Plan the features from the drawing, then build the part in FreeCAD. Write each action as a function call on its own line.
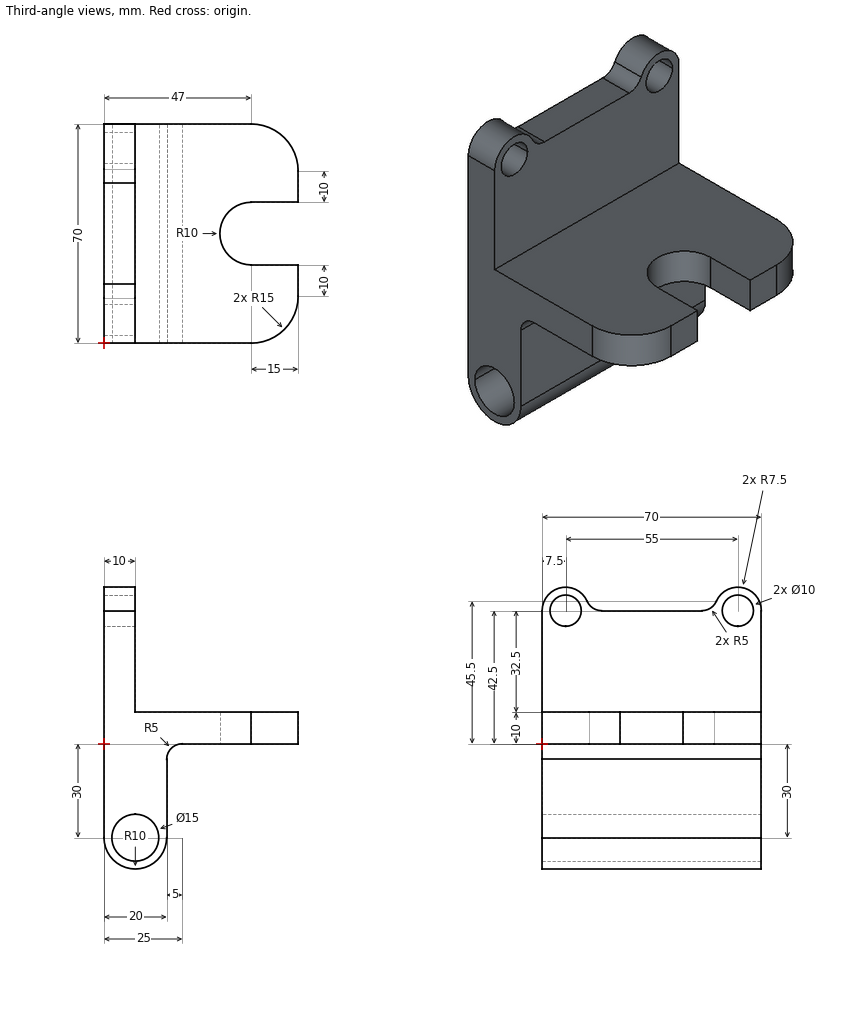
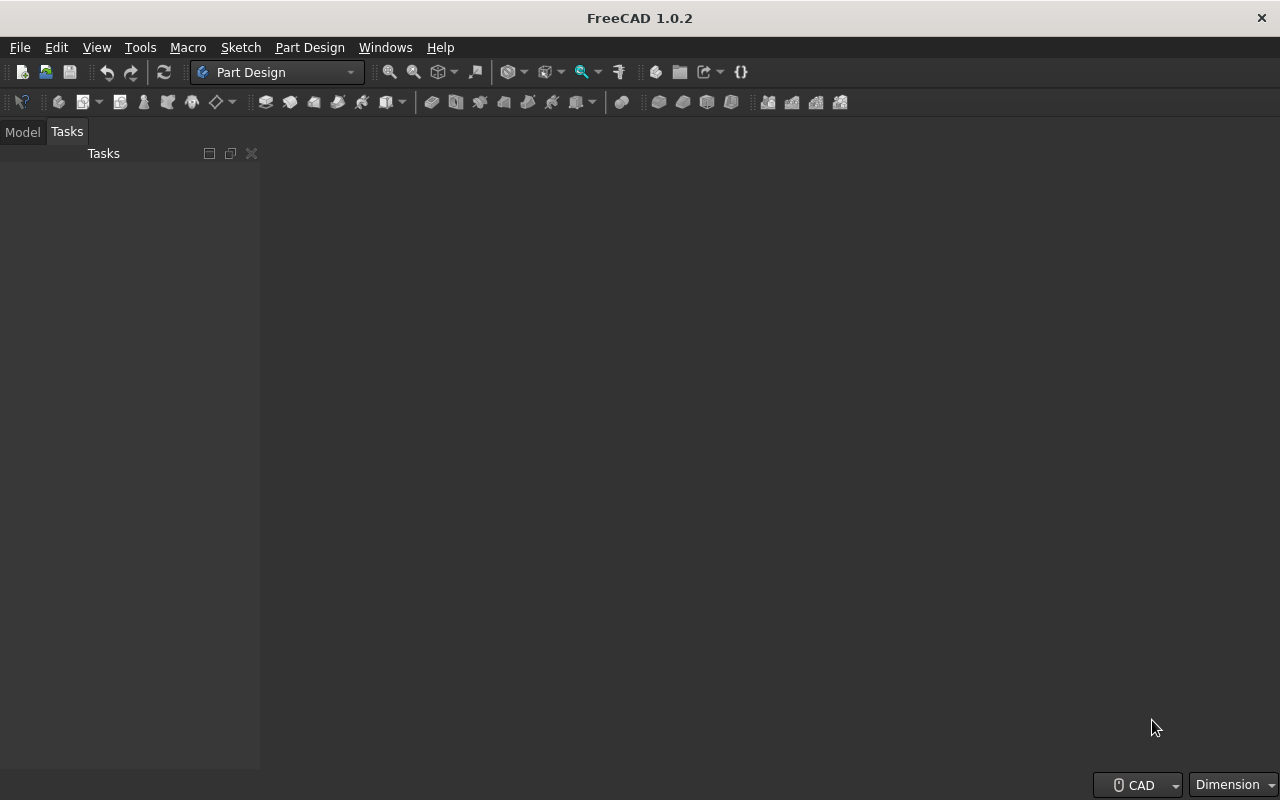
click(22, 72)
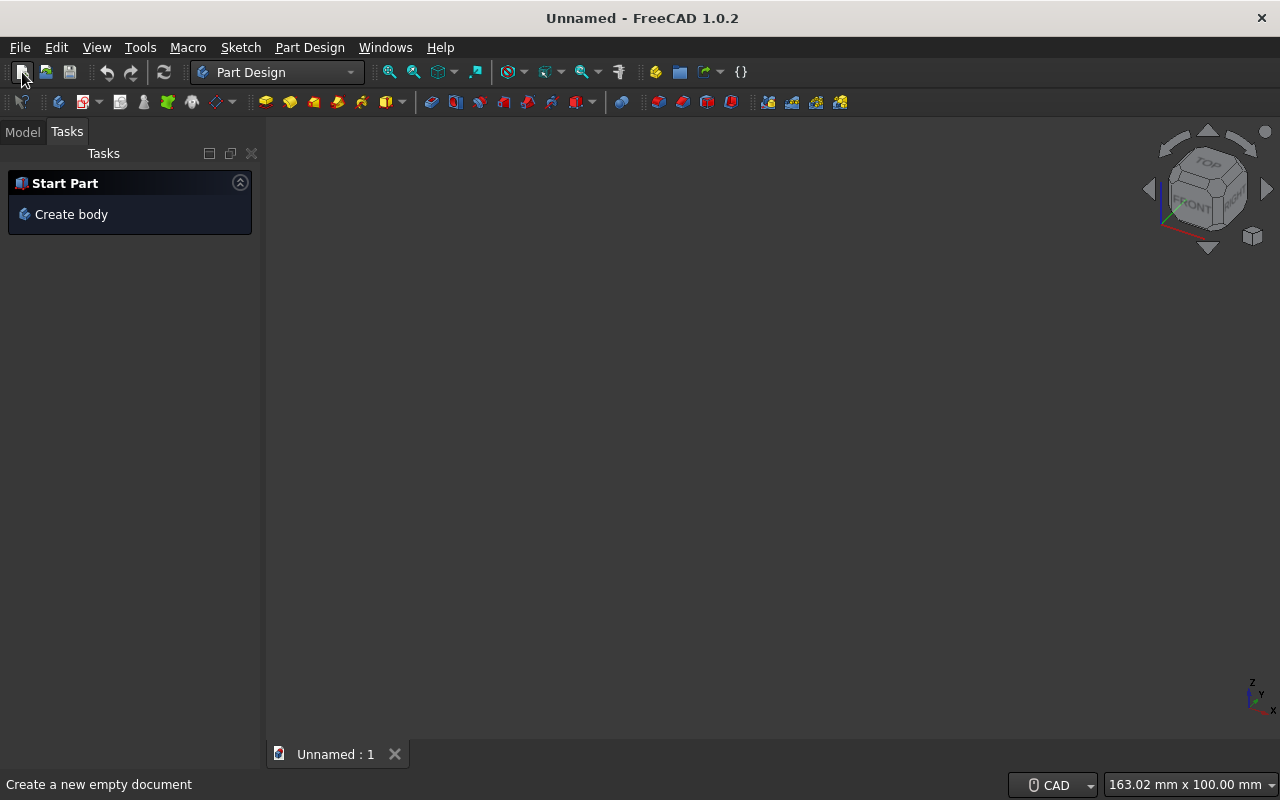
click(84, 102)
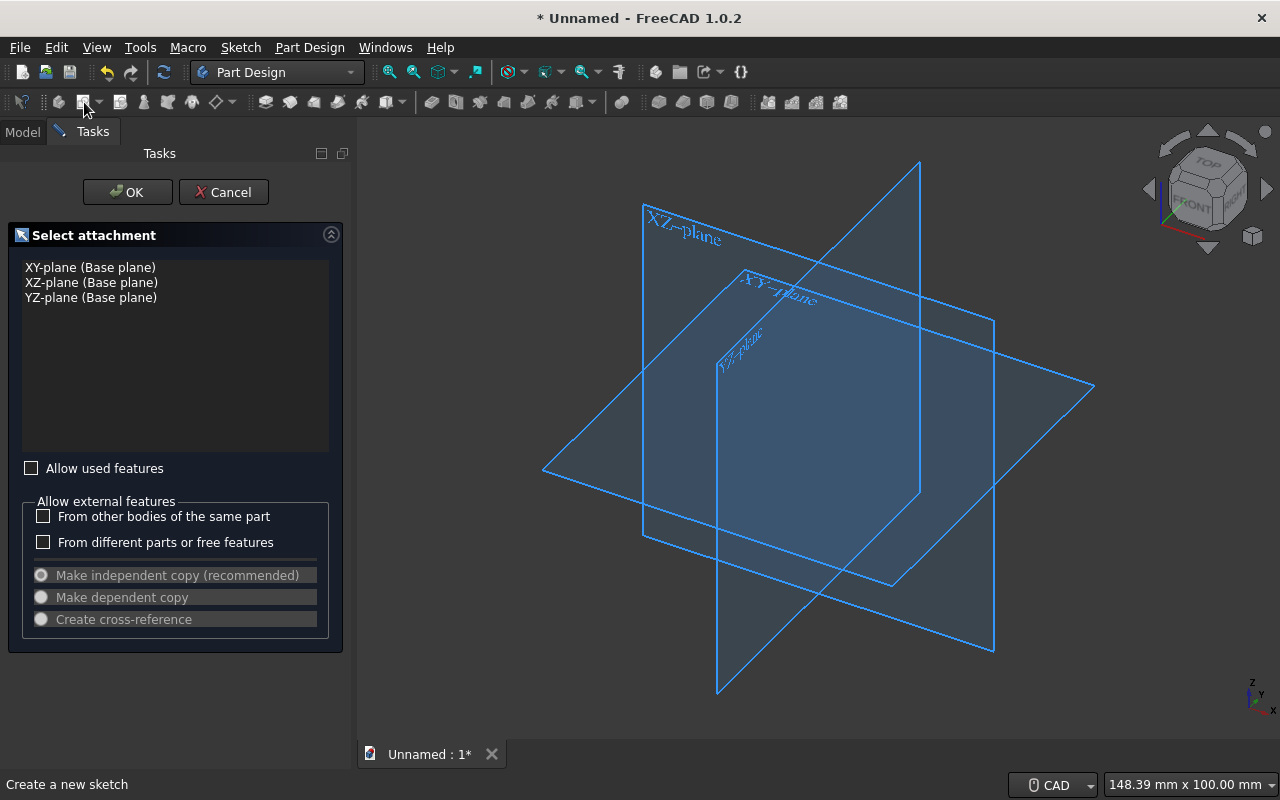
click(82, 268)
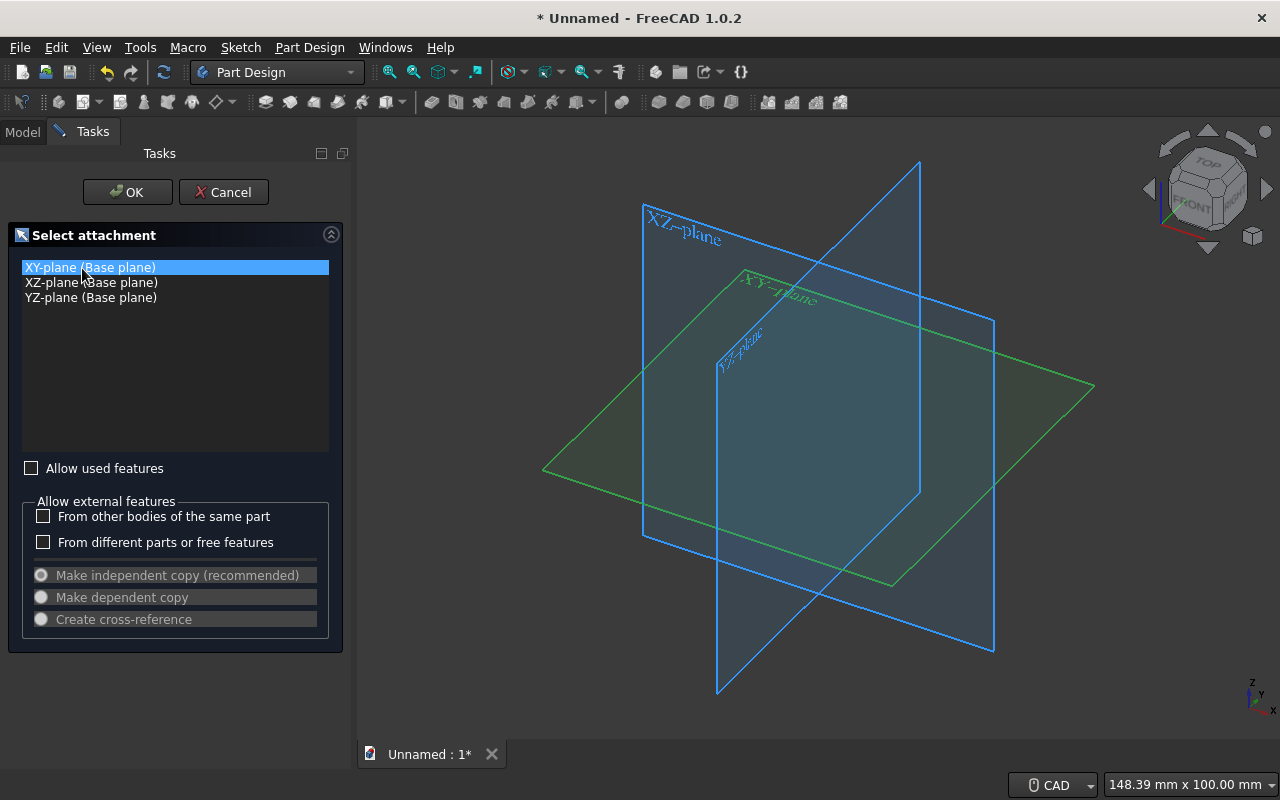
click(128, 192)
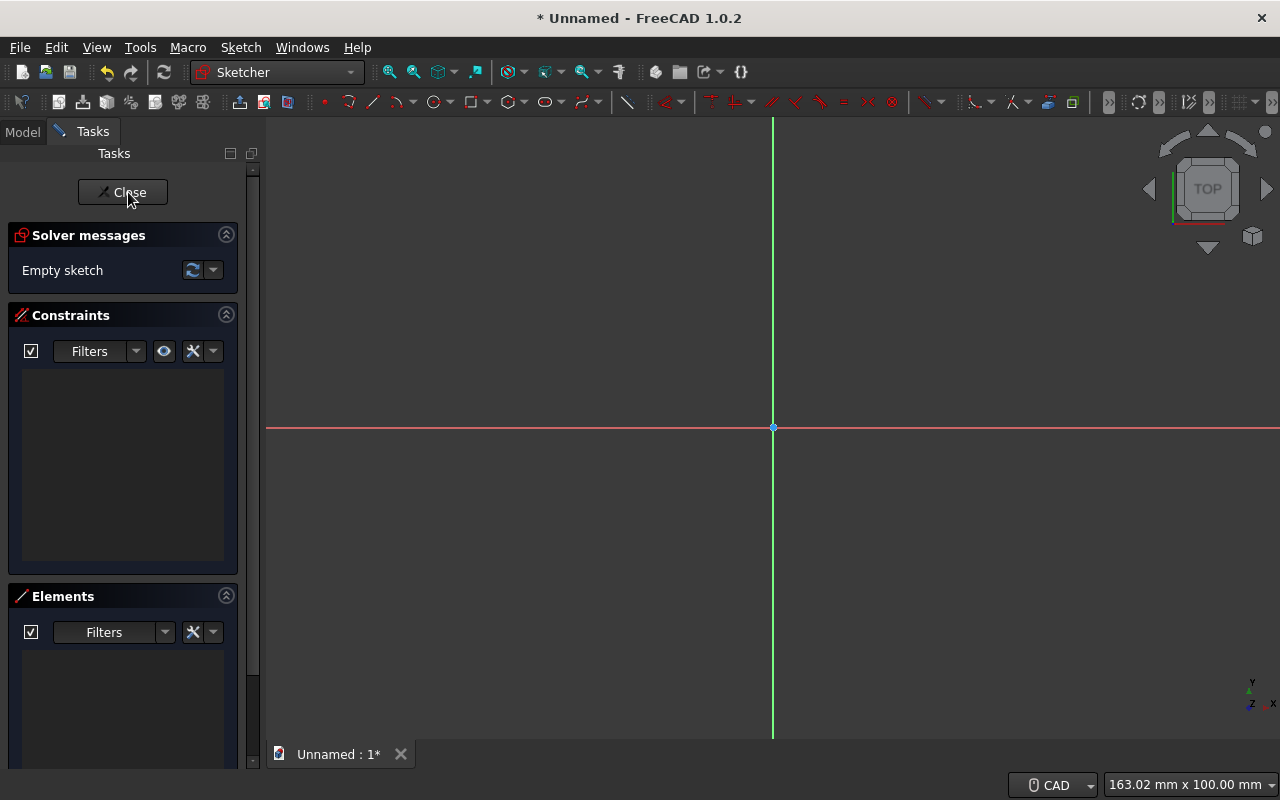
scroll(294, 711, down, 2)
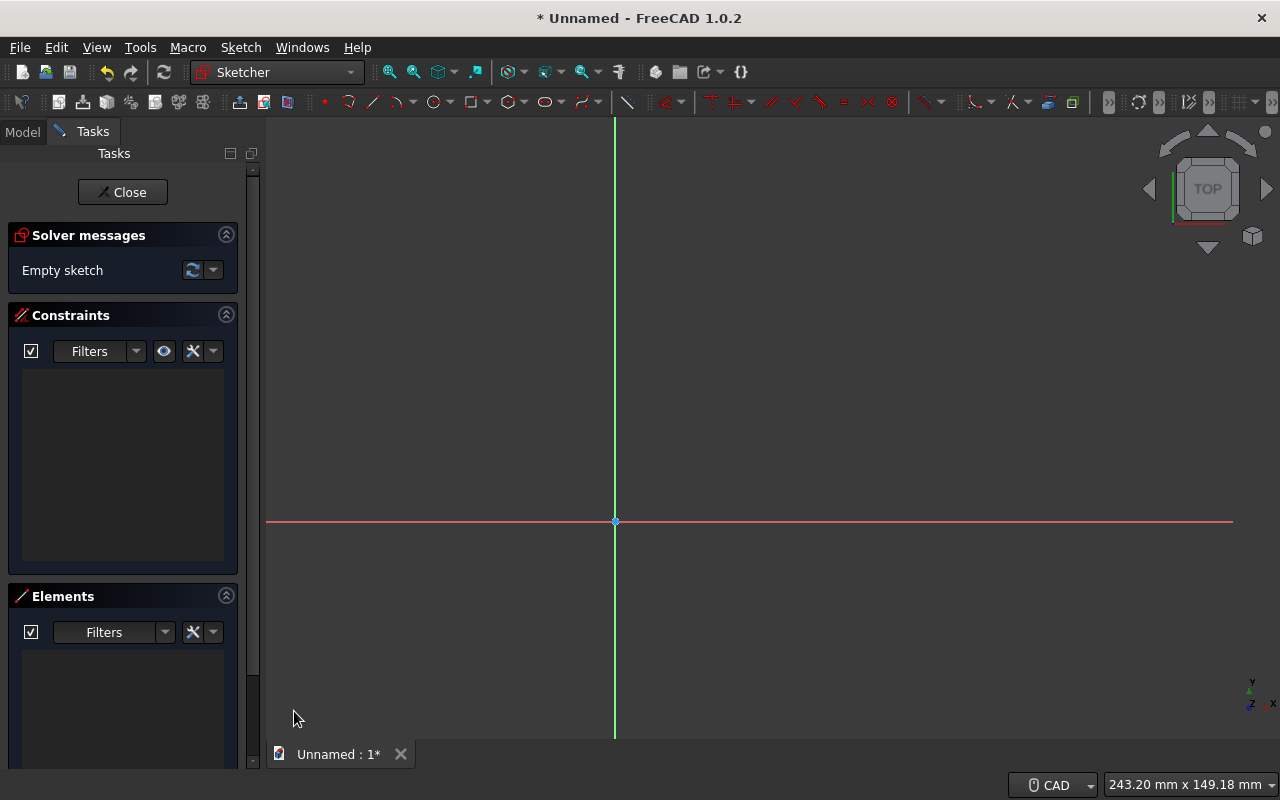
scroll(825, 269, up, 2)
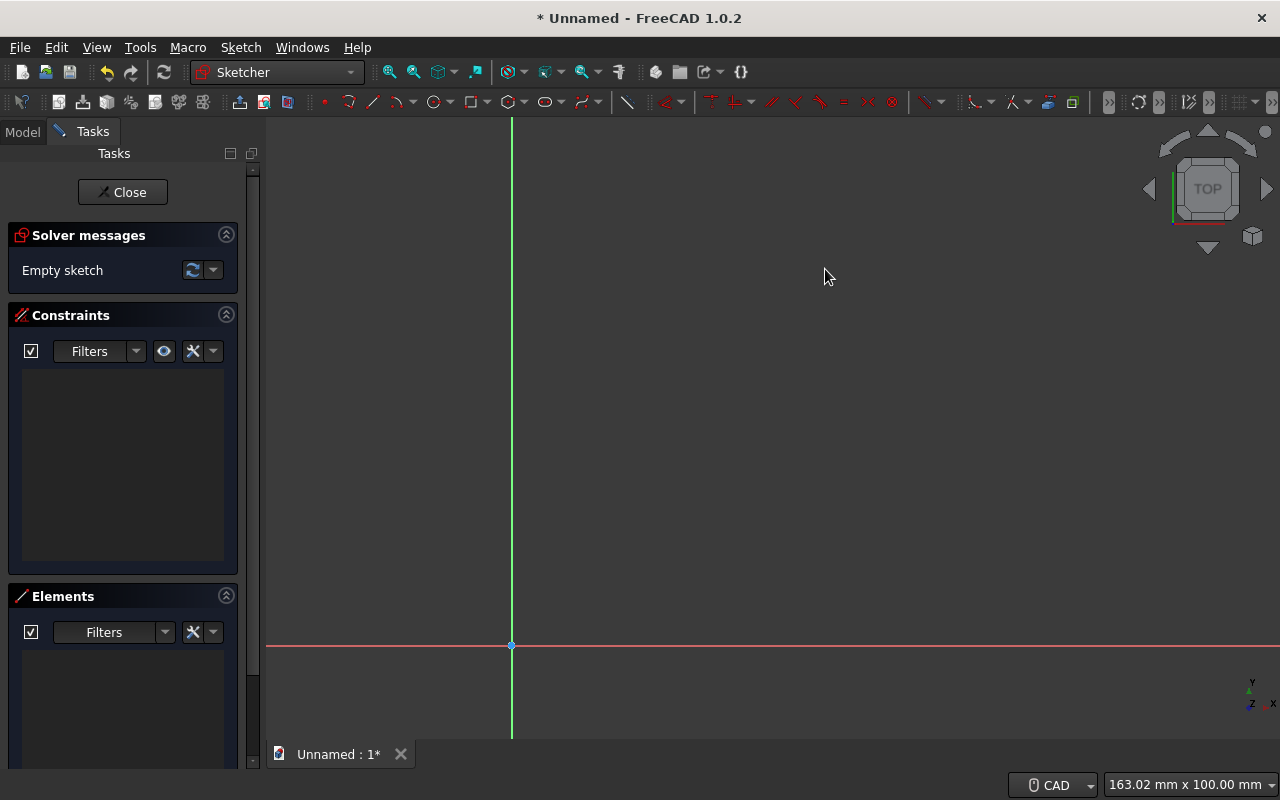
click(350, 102)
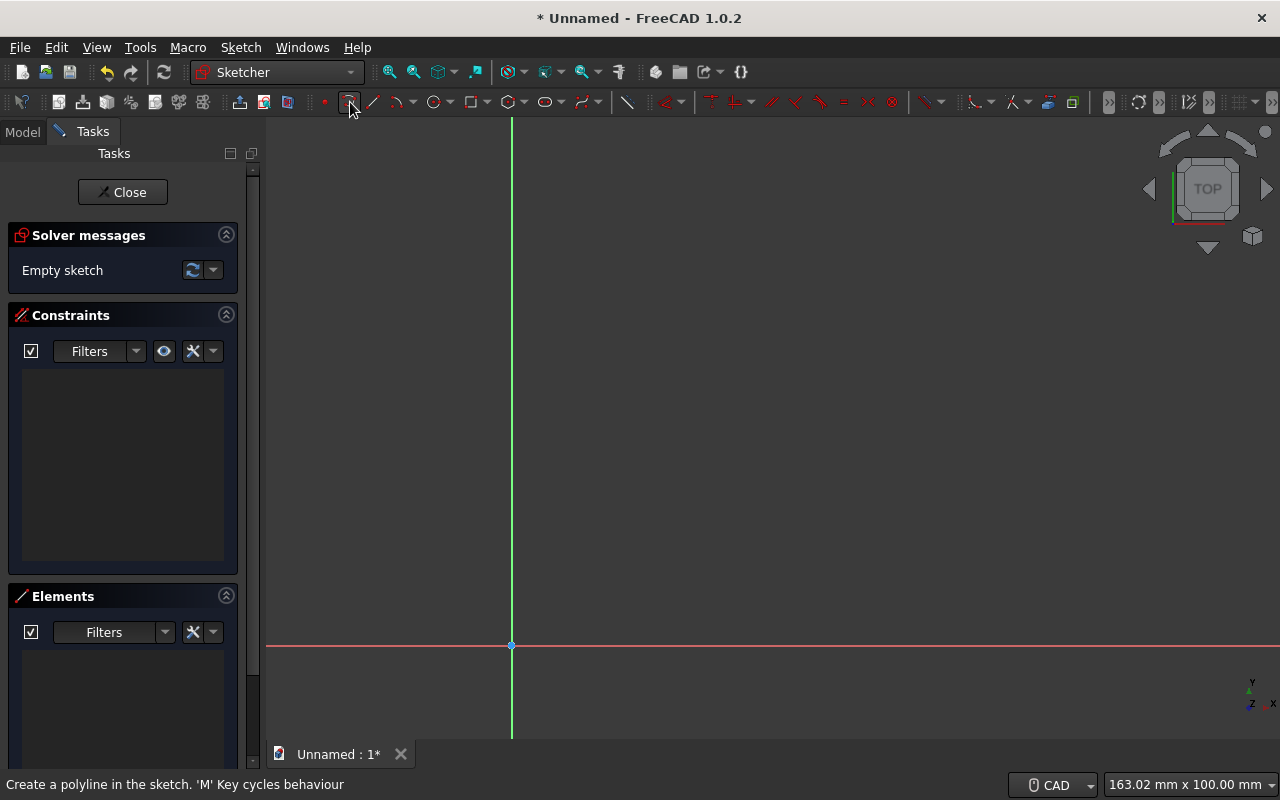
click(897, 552)
click(897, 490)
click(804, 490)
right_click(804, 490)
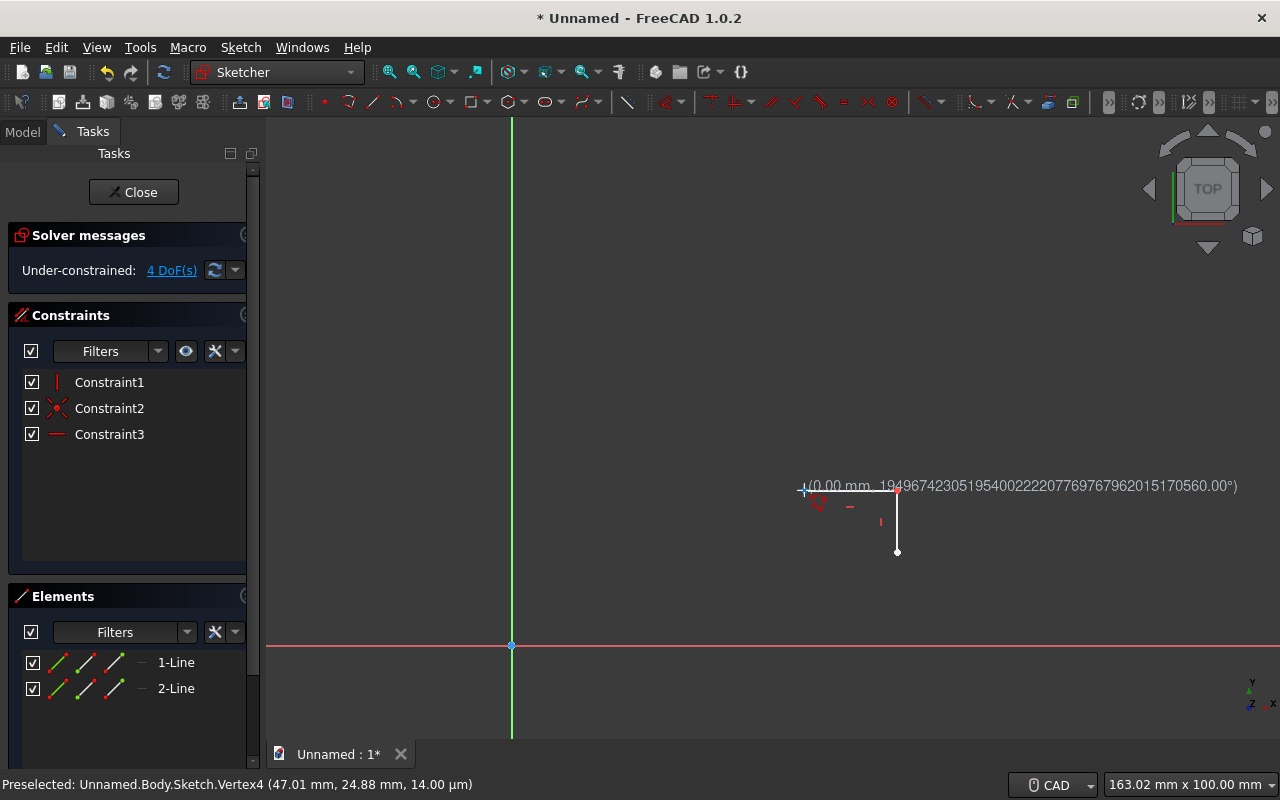
click(804, 366)
click(897, 366)
click(897, 304)
right_click(897, 304)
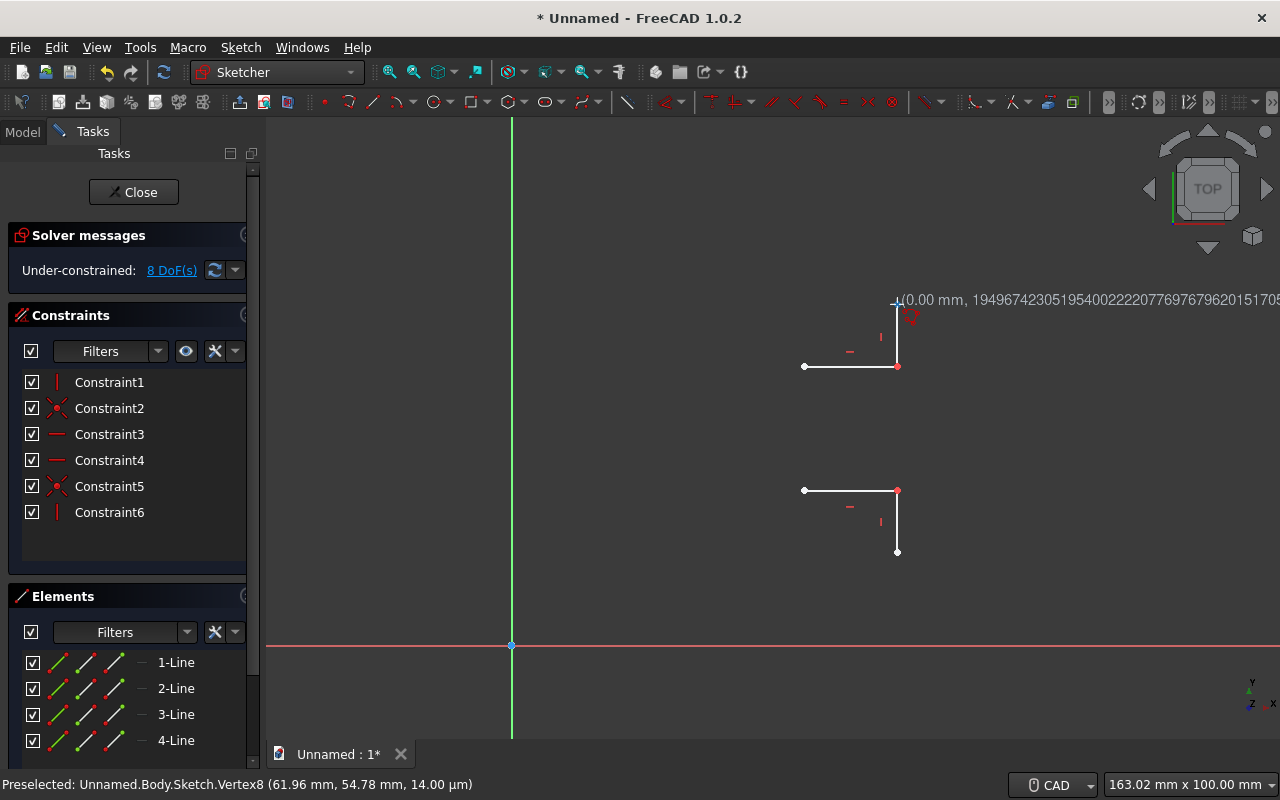
click(804, 210)
click(512, 210)
click(512, 646)
click(804, 637)
right_click(804, 637)